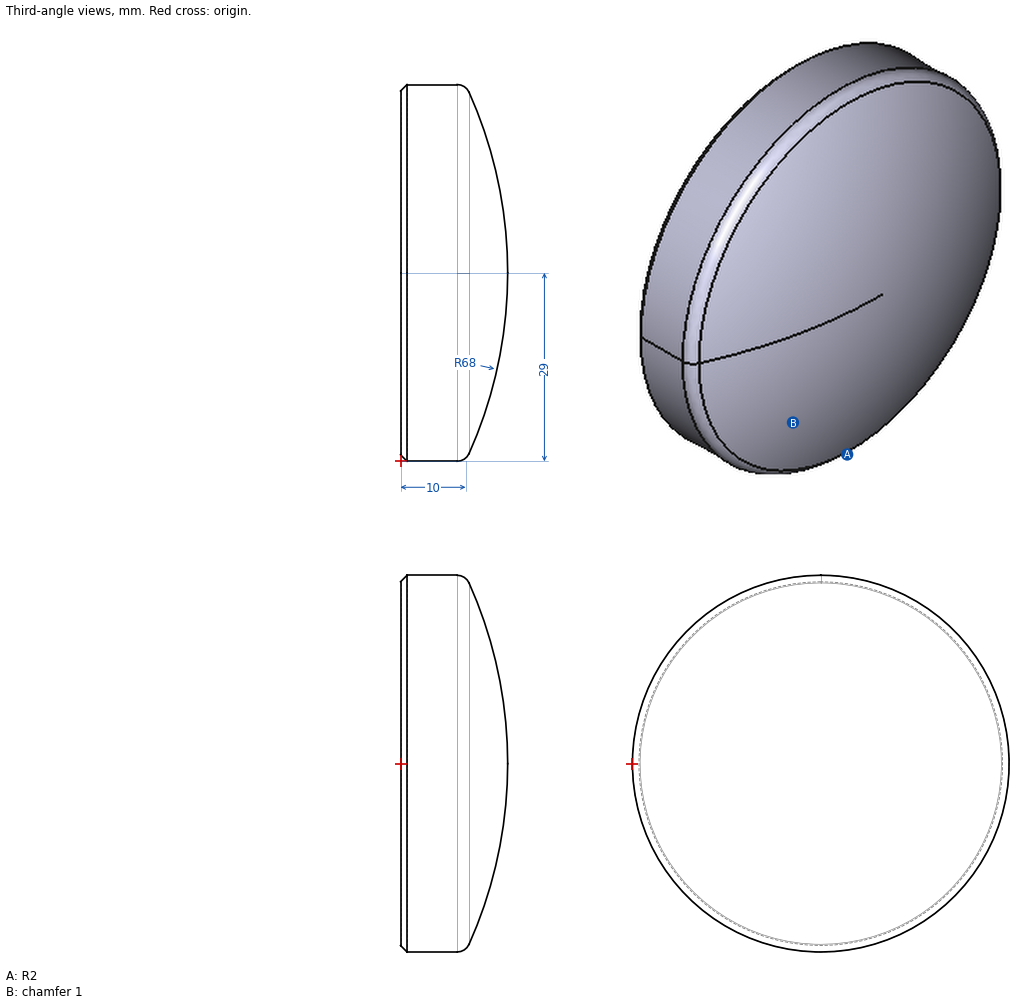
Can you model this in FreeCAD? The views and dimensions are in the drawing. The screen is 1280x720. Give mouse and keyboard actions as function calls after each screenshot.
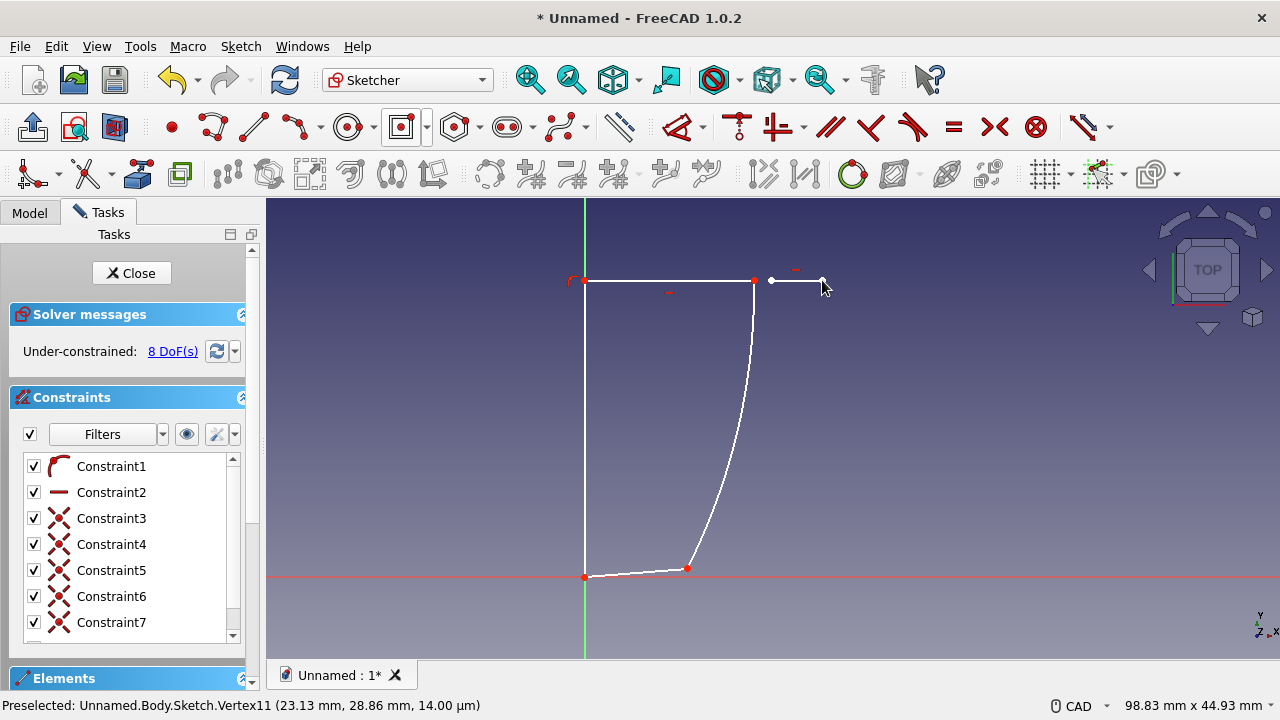
click(786, 281)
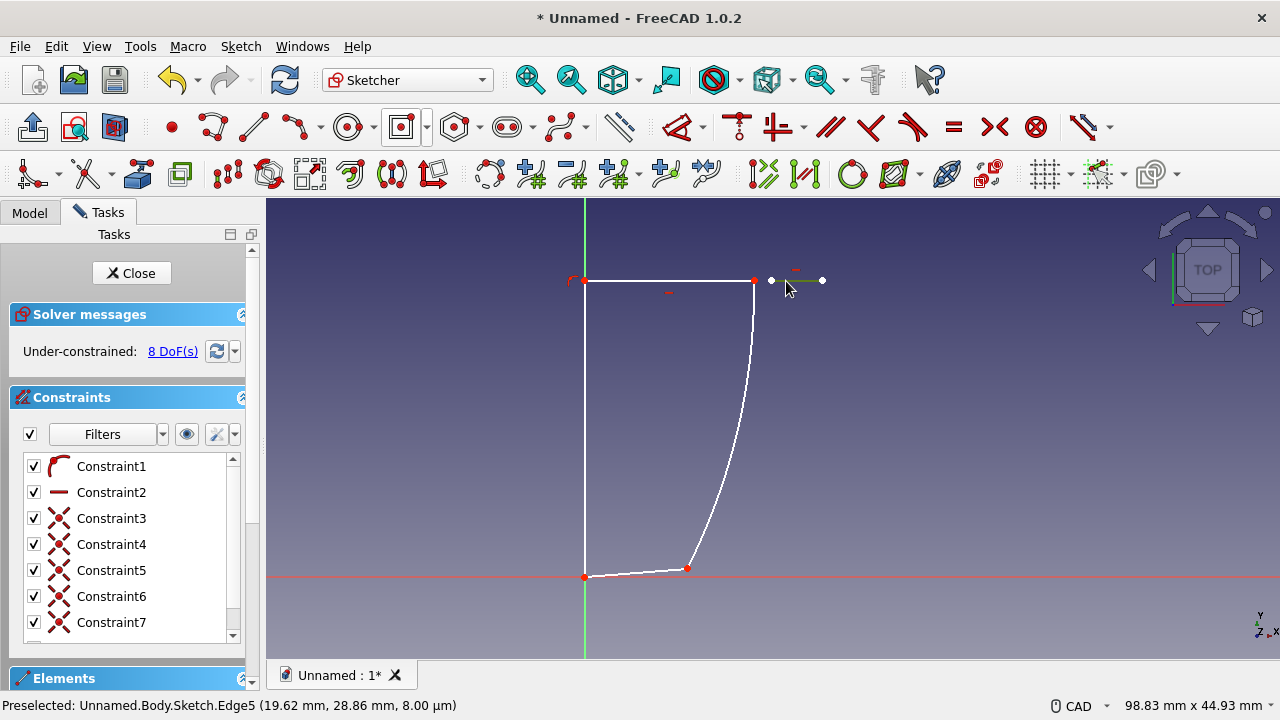
click(620, 128)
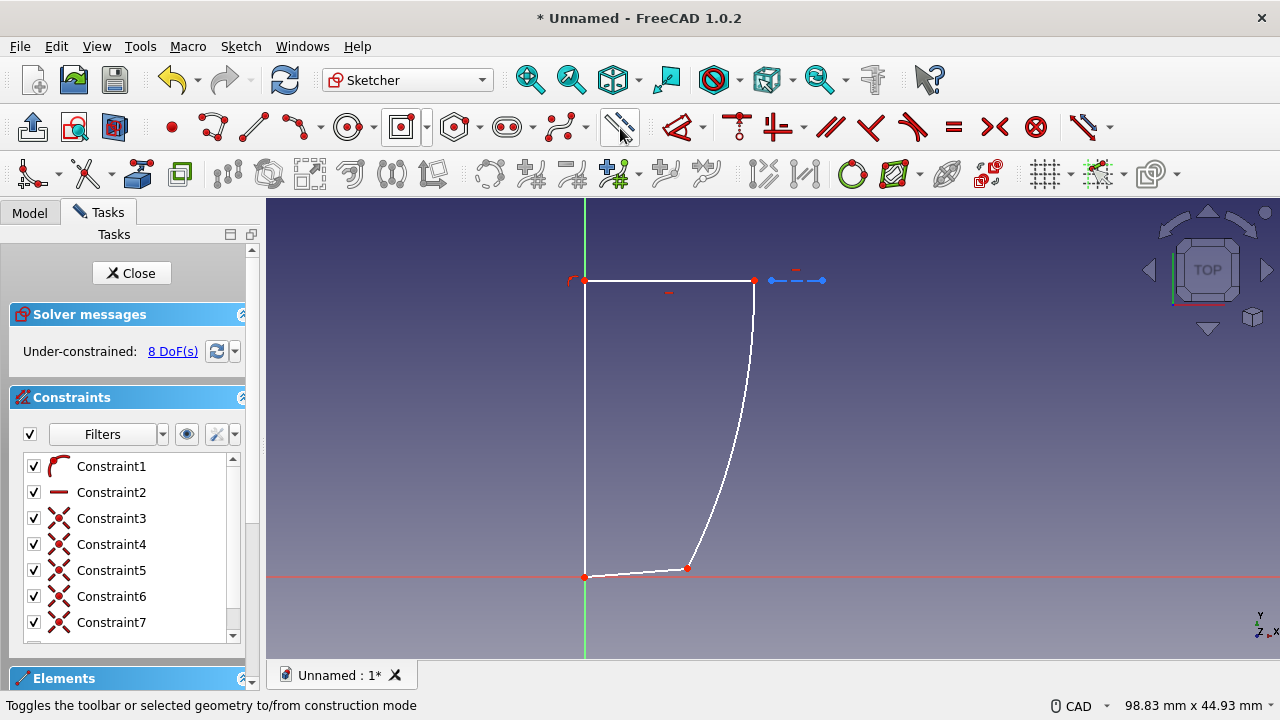
click(615, 575)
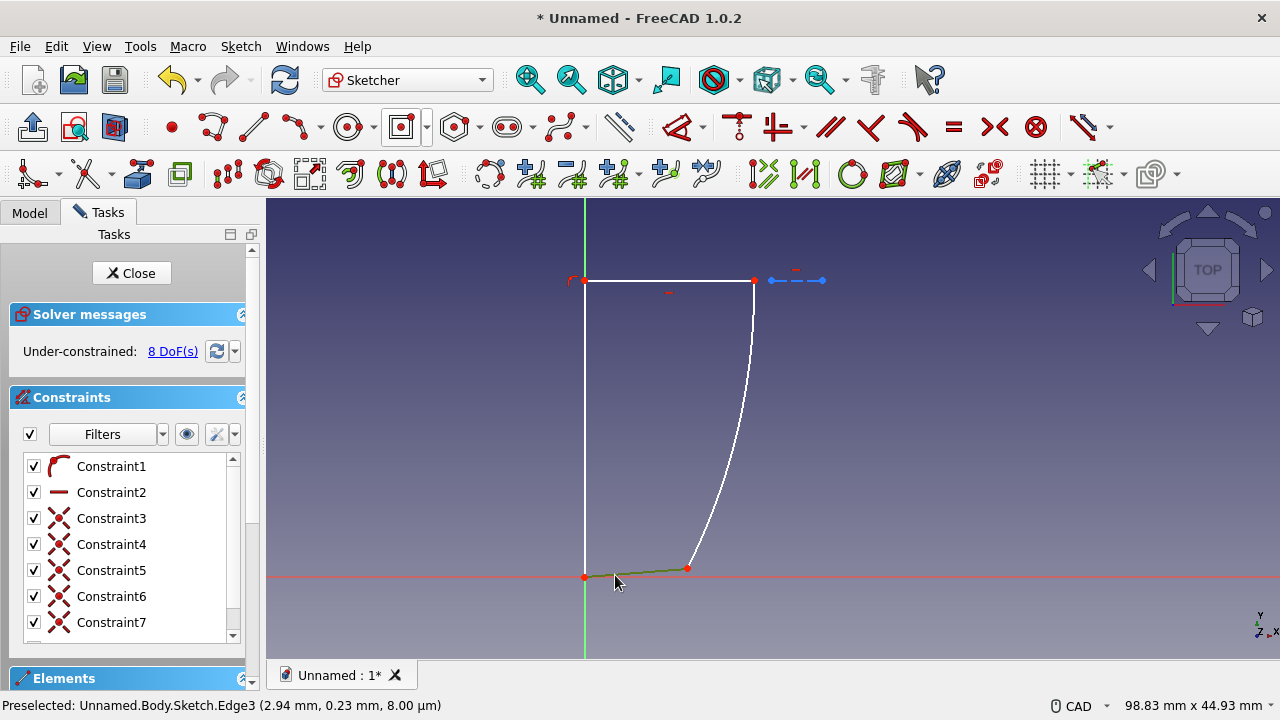
key(h)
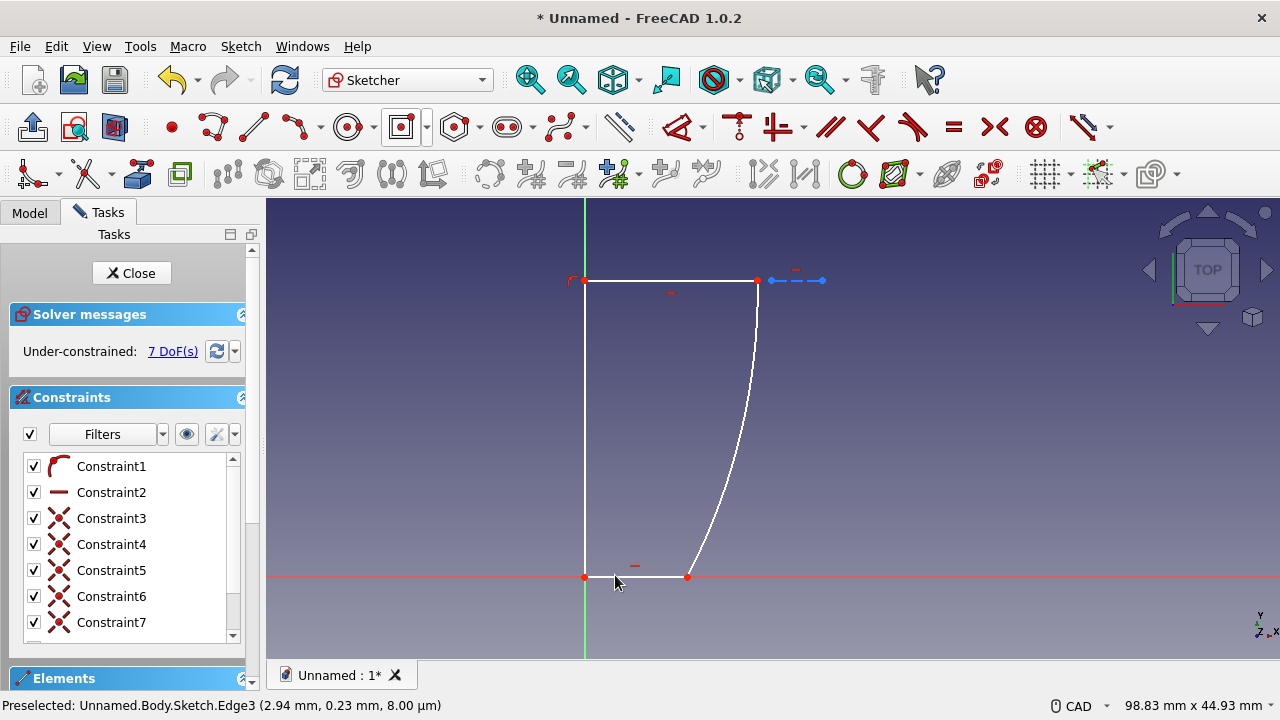
click(723, 492)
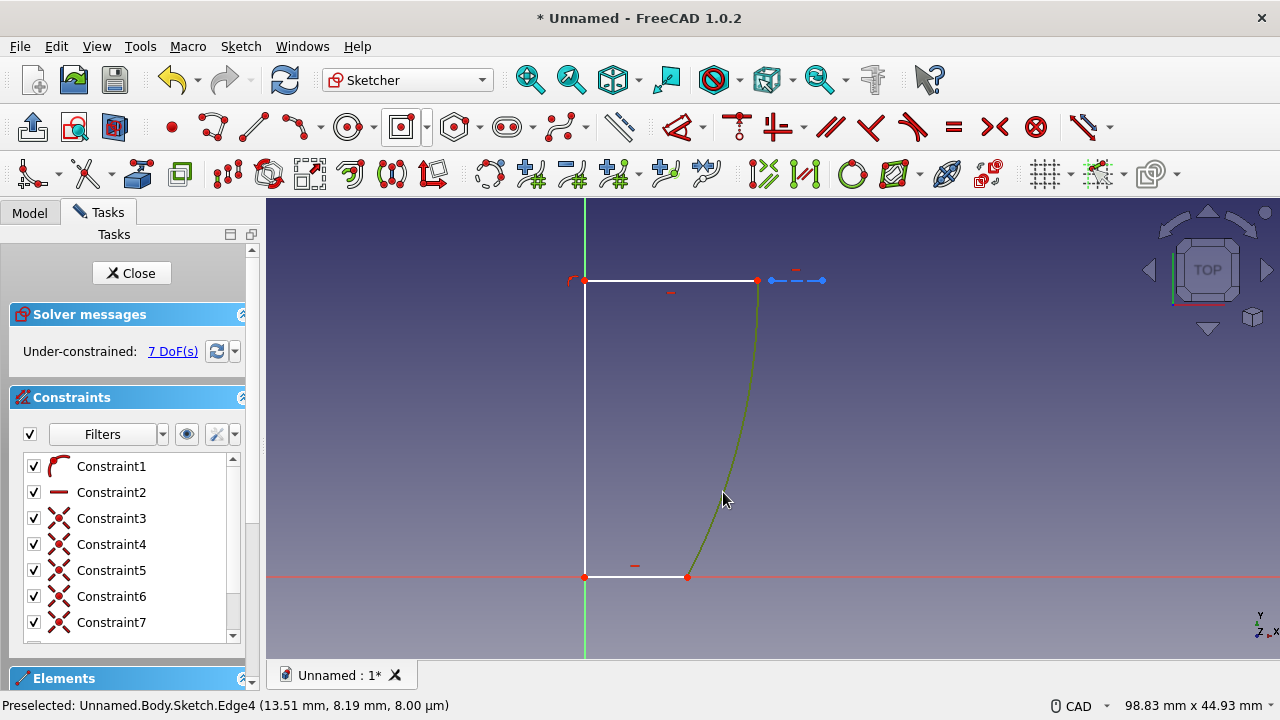
click(702, 128)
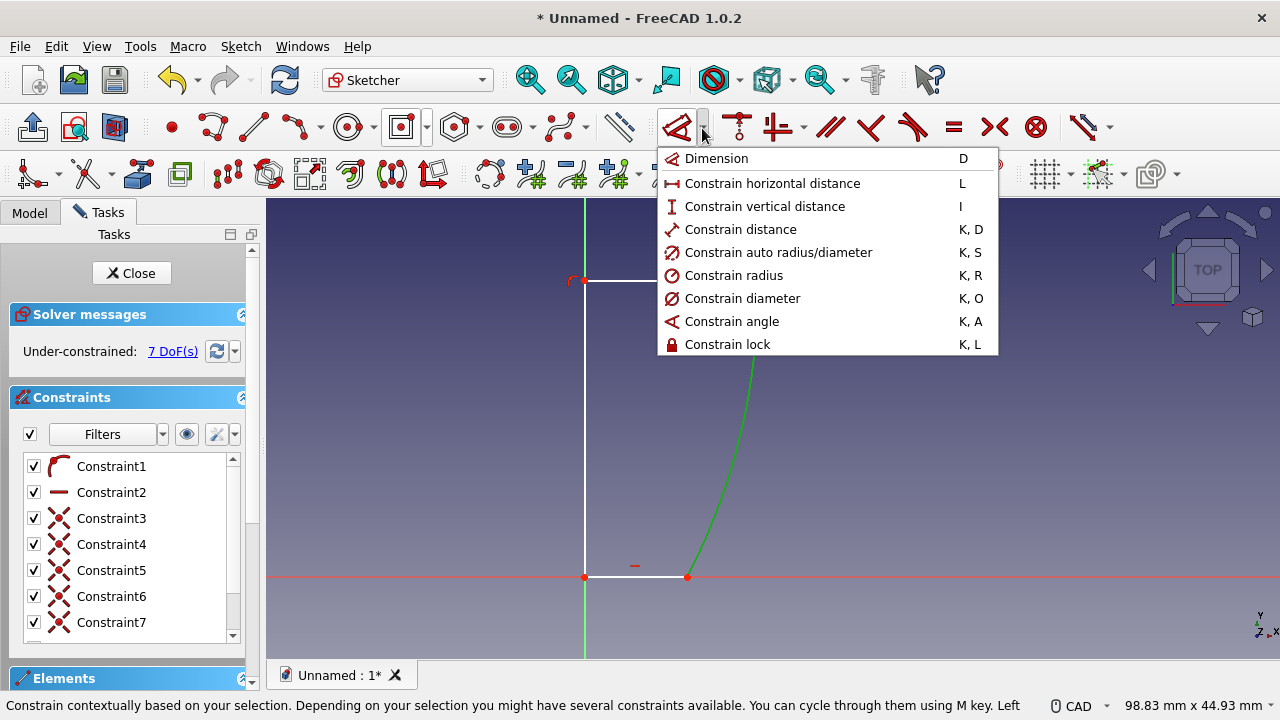
click(828, 276)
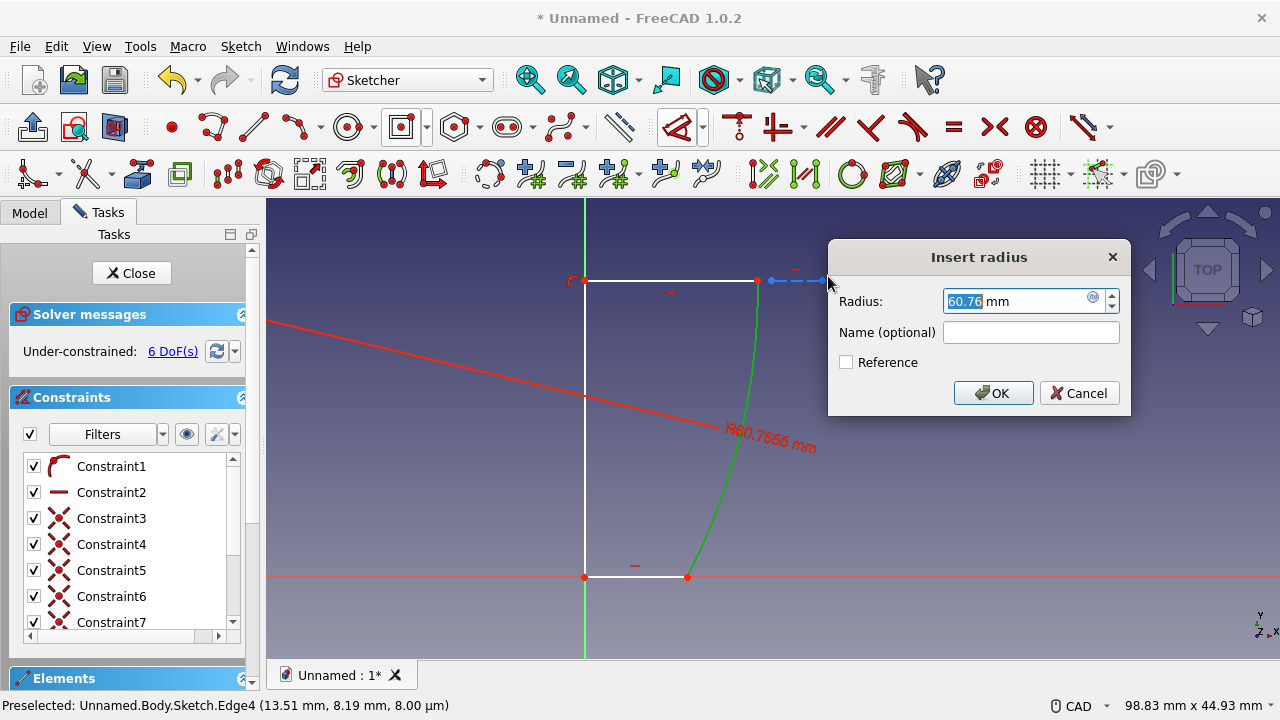
text(68)
key(Return)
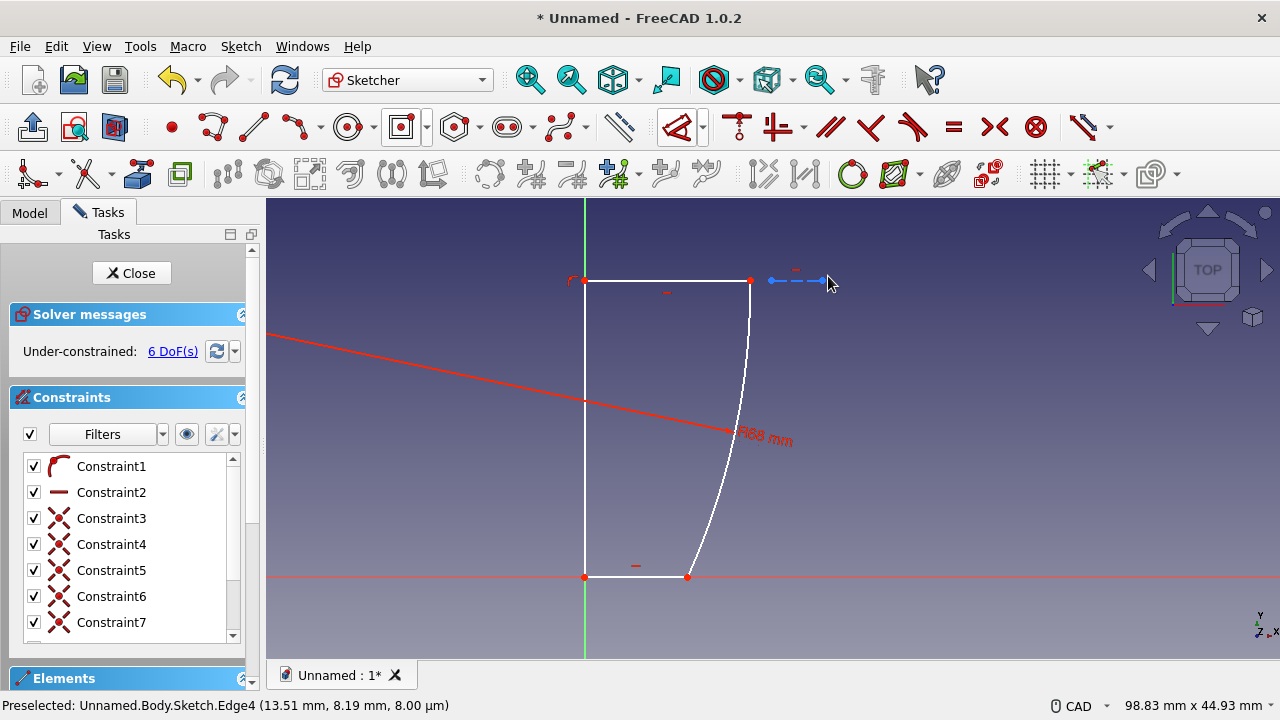
click(585, 370)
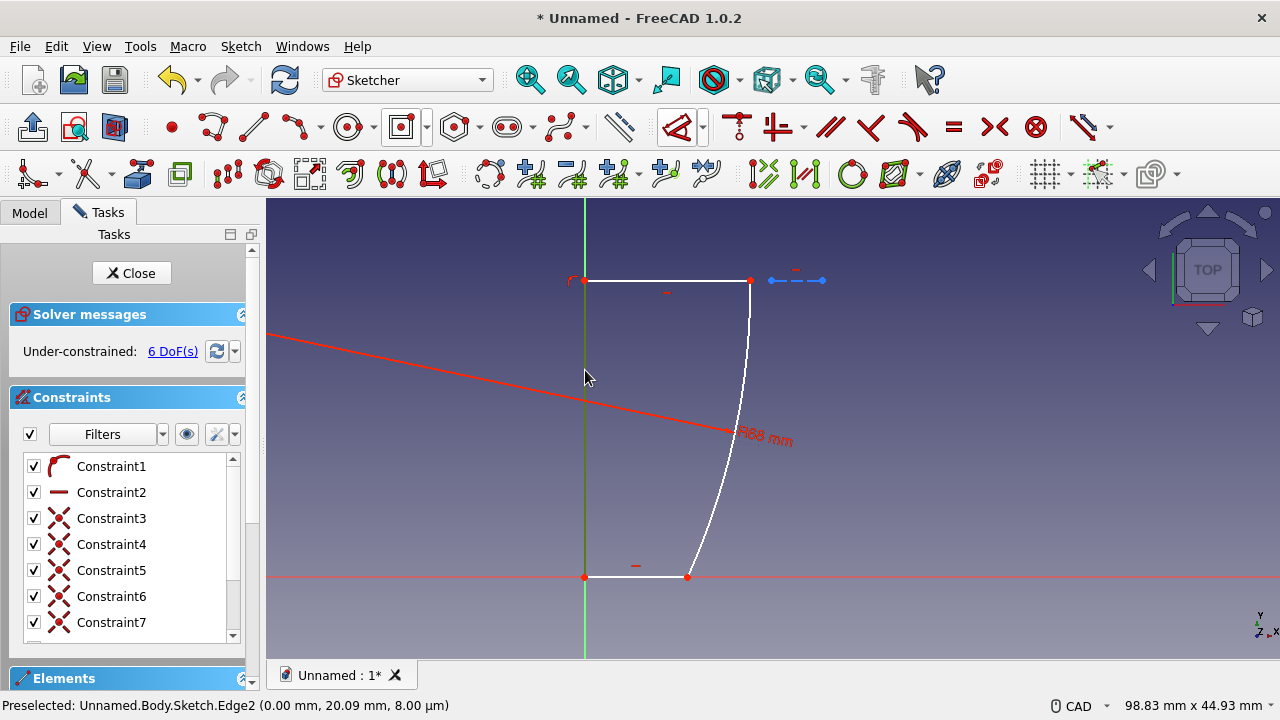
click(702, 128)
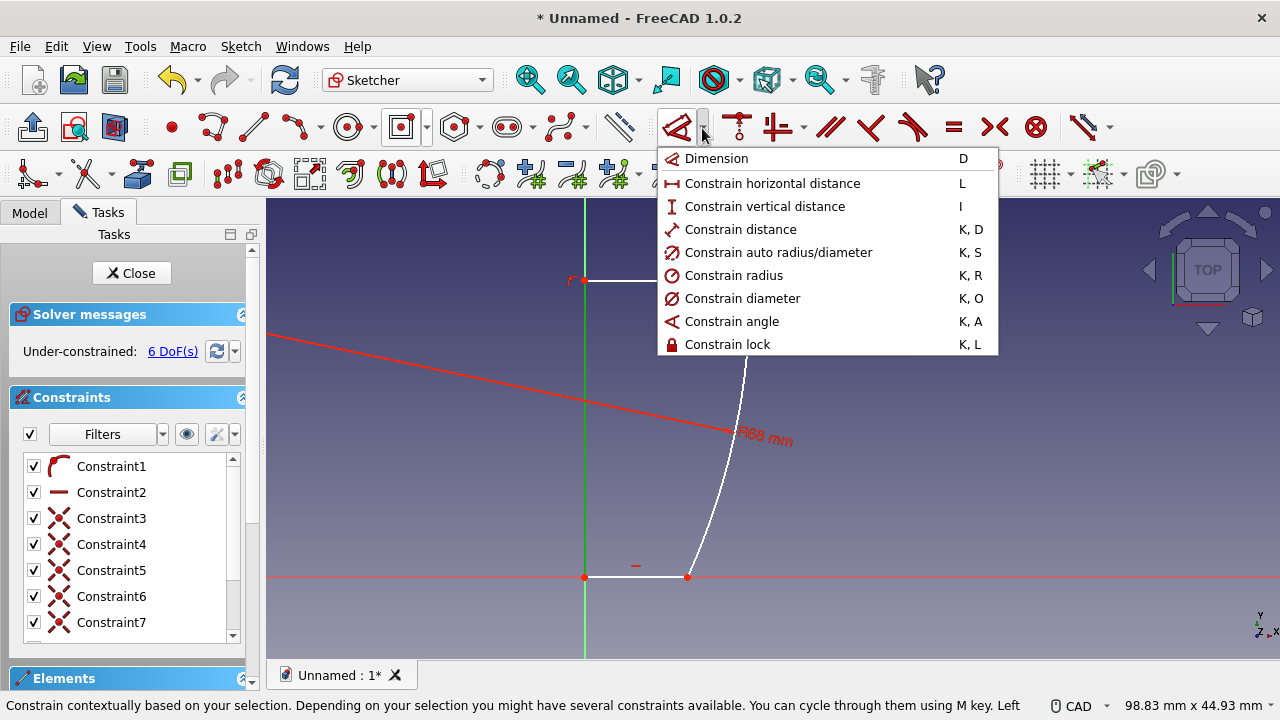
click(828, 206)